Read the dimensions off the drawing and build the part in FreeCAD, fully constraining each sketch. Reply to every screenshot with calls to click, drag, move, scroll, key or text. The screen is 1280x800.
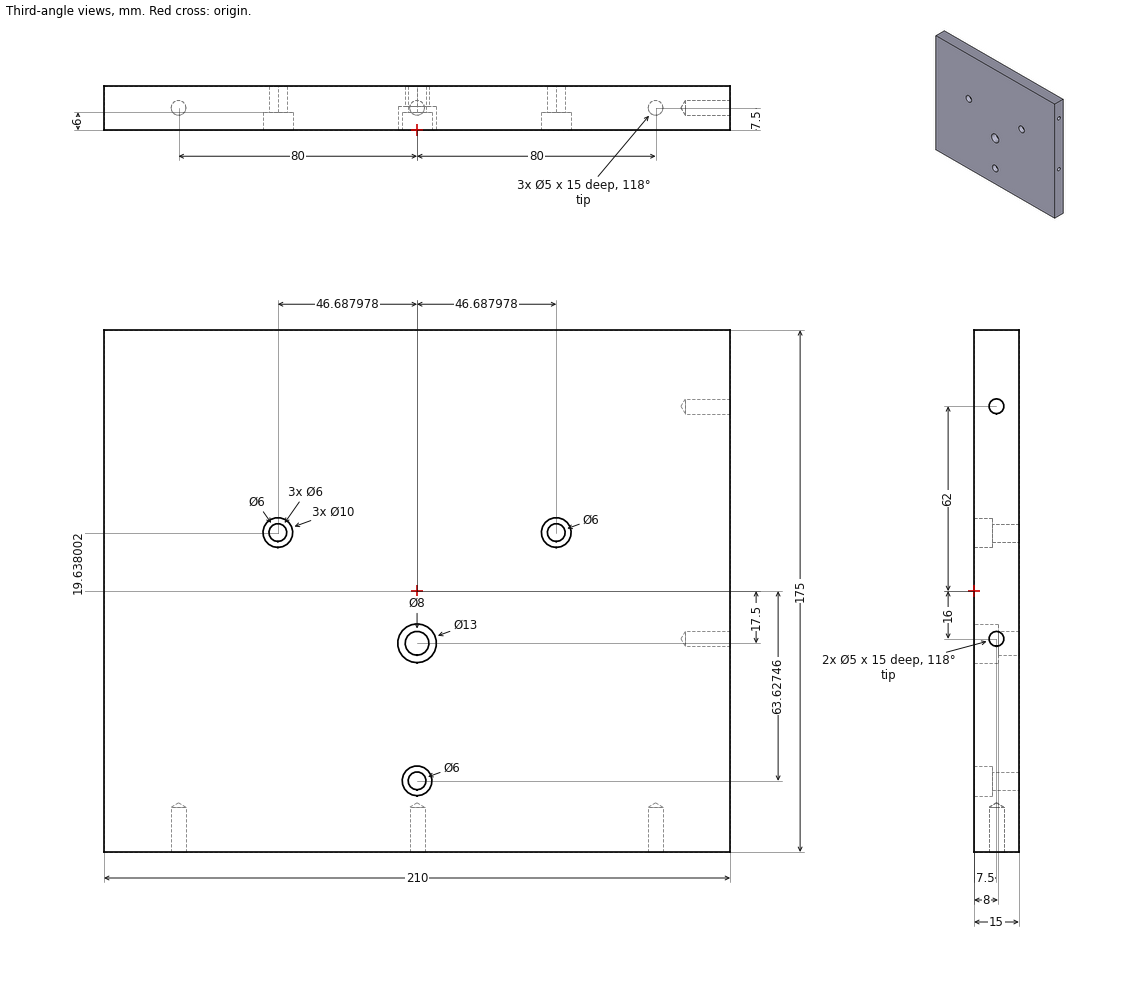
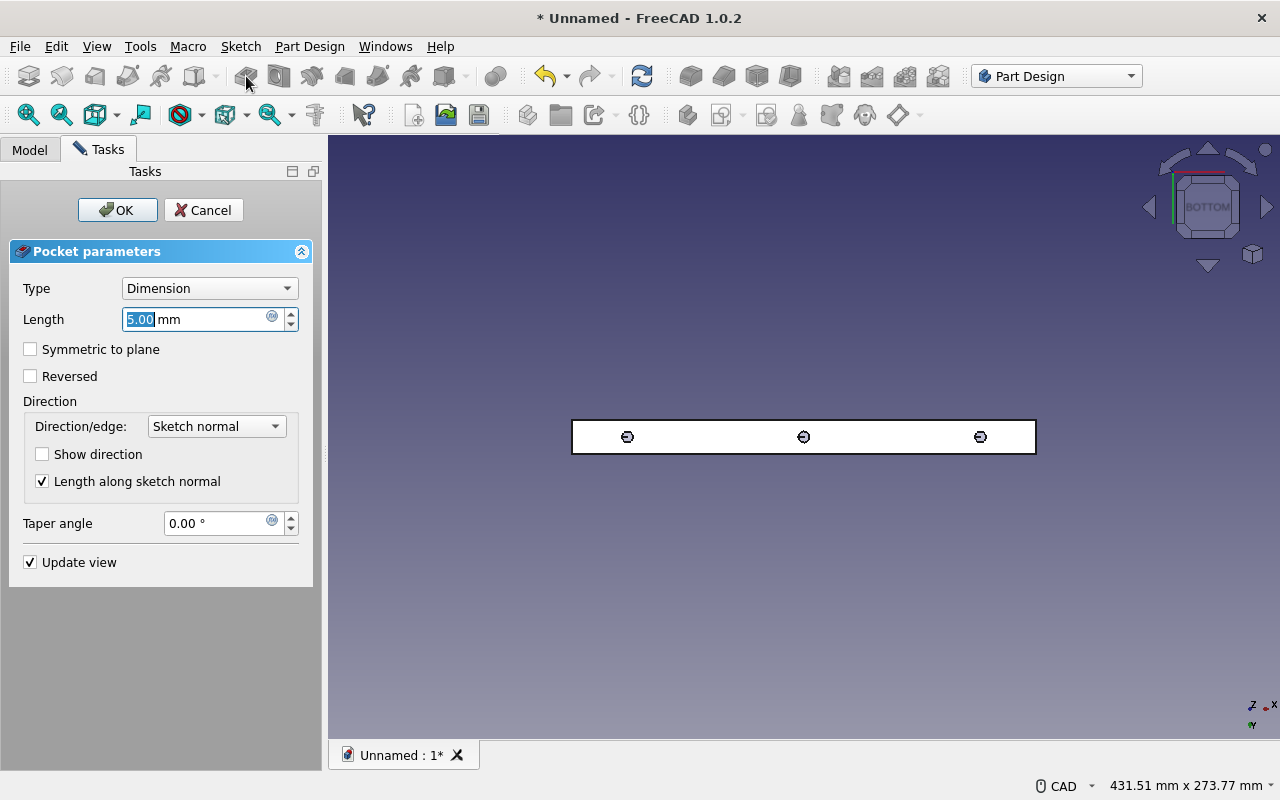
text(8)
key(Tab)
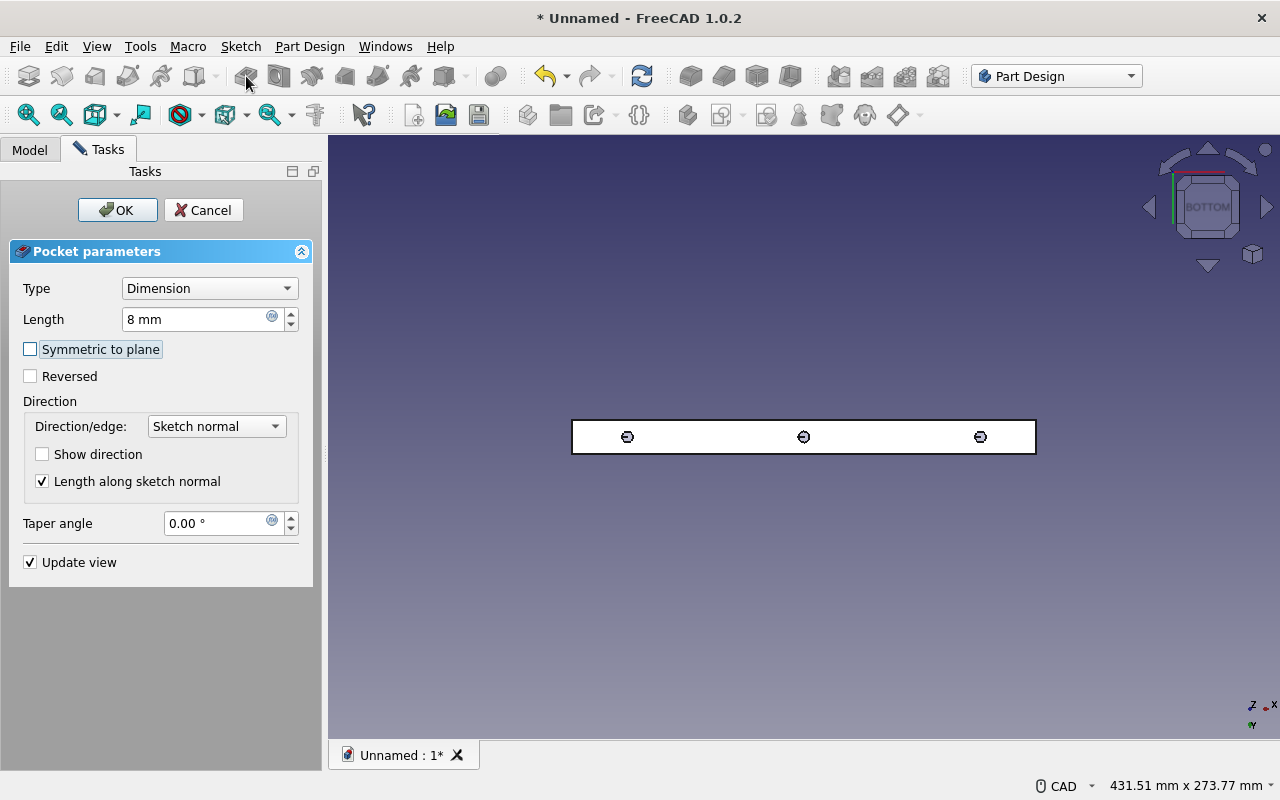
click(118, 210)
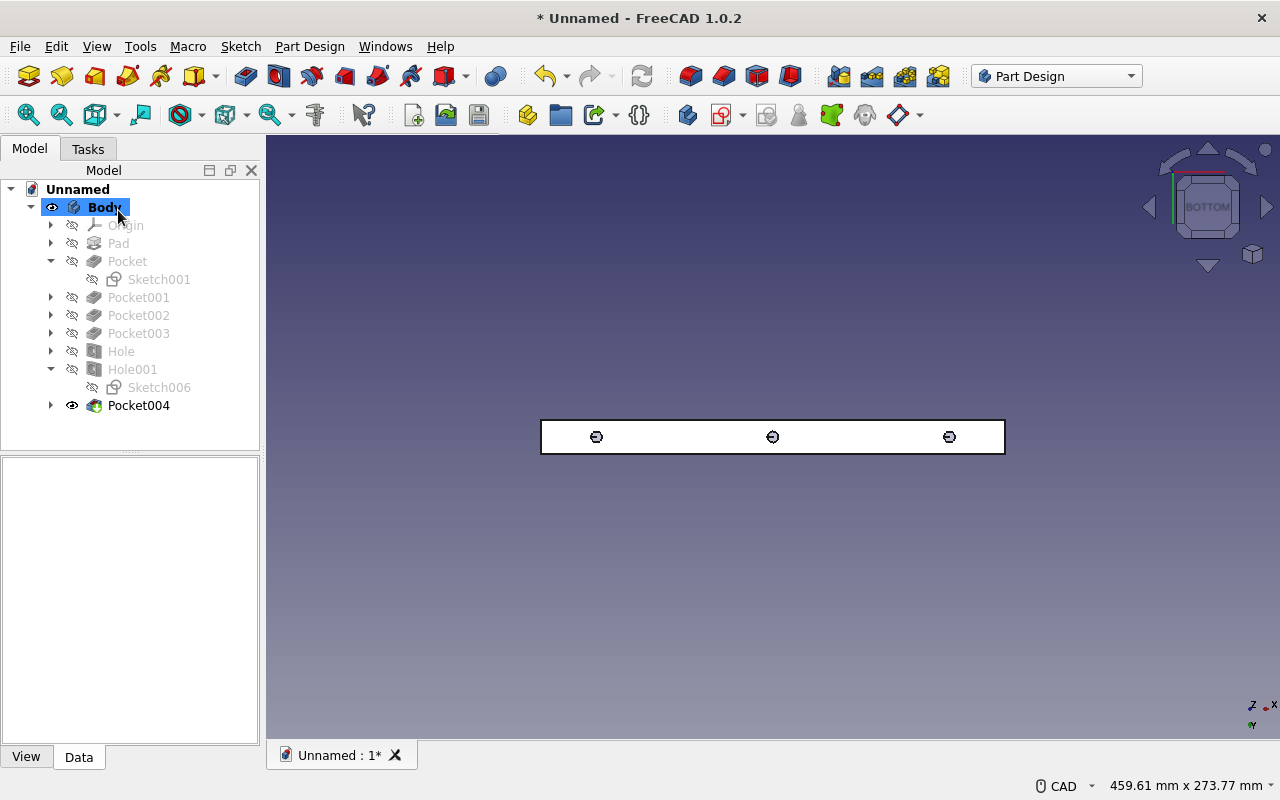
click(720, 116)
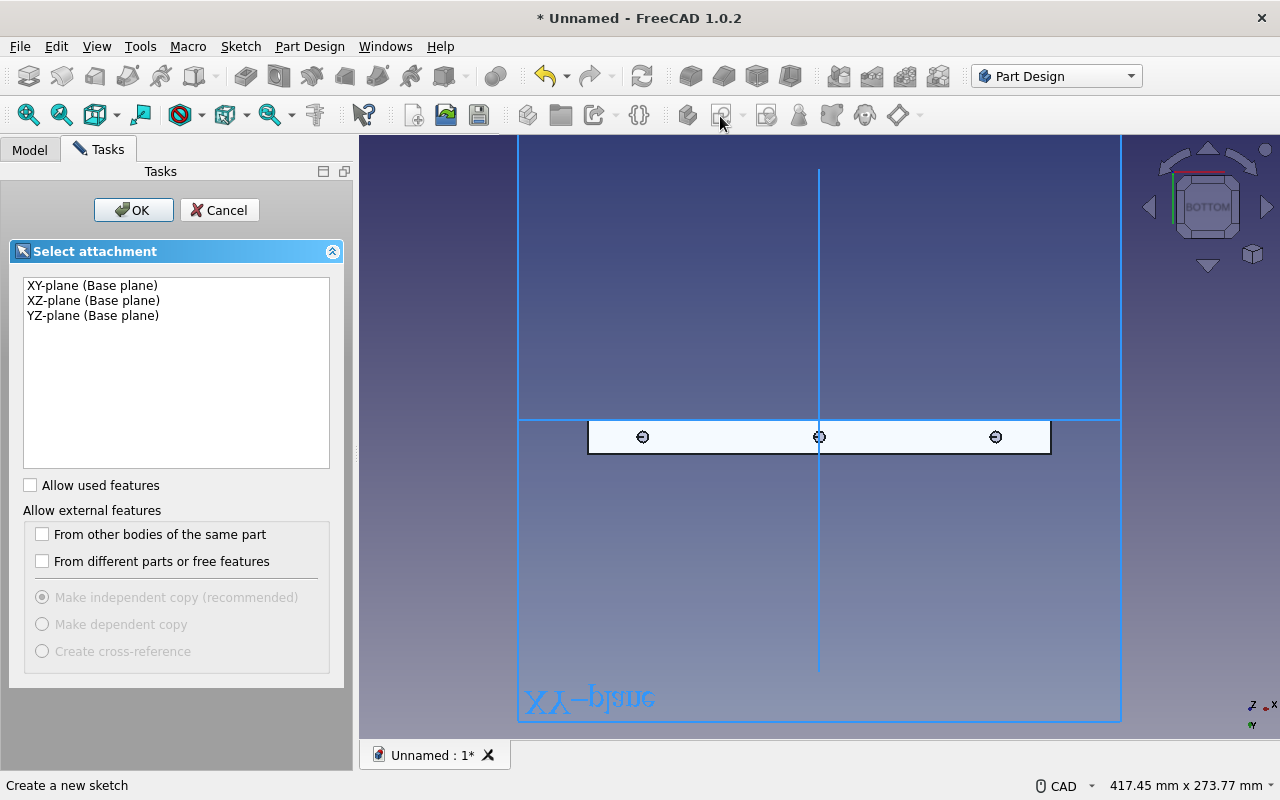
click(84, 300)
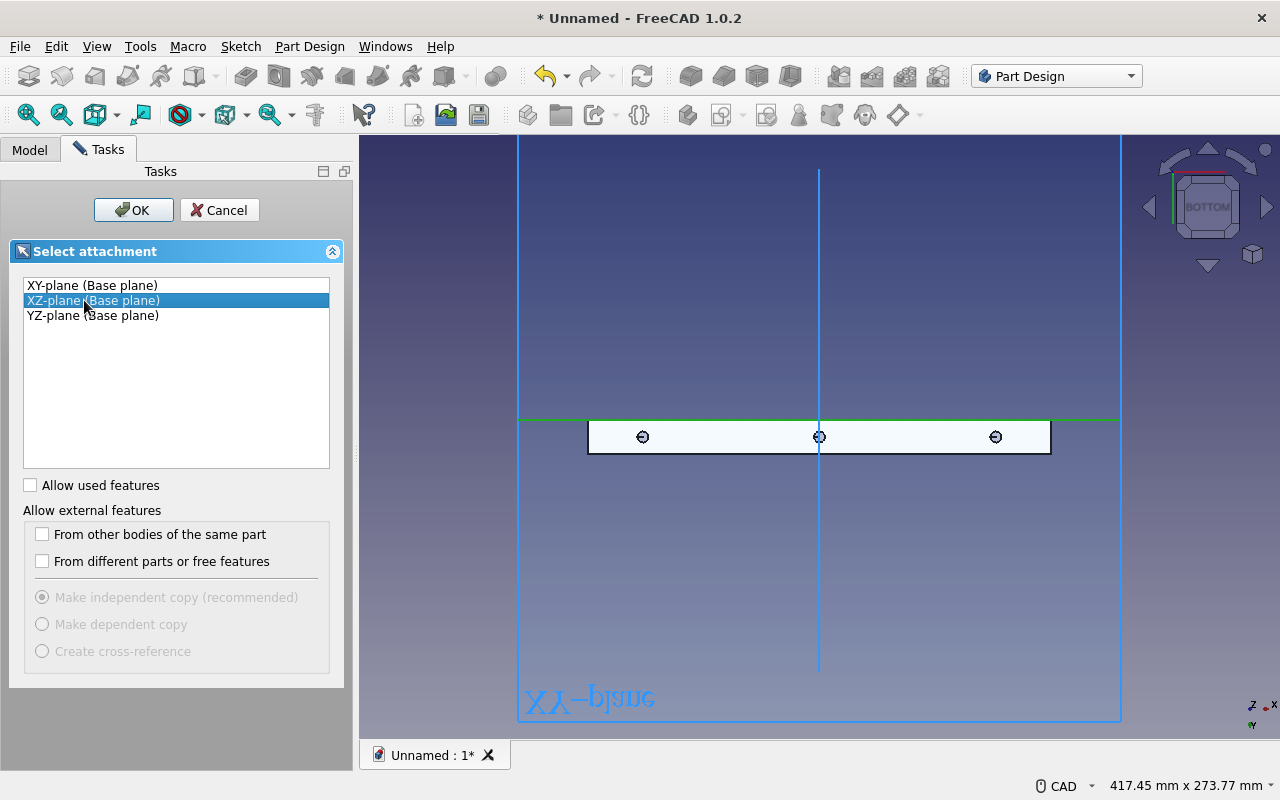
click(134, 210)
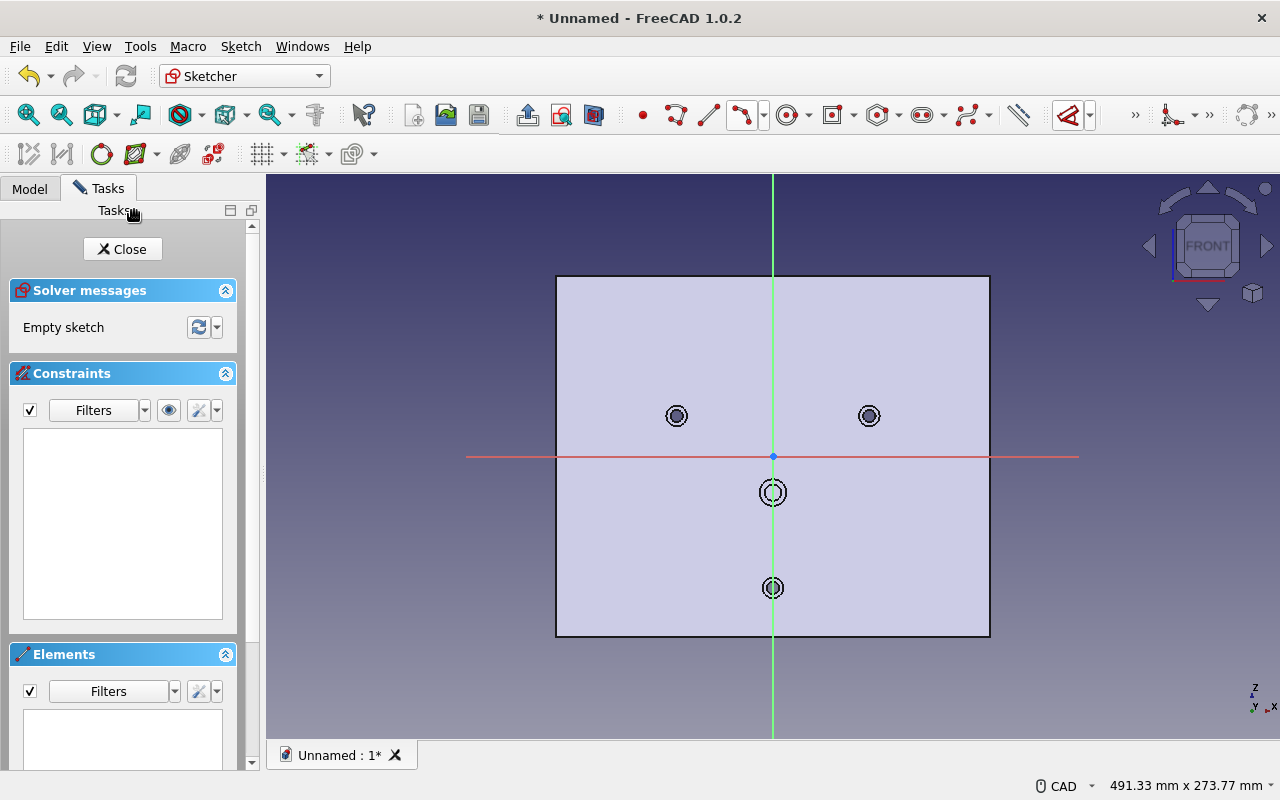
scroll(777, 495, up, 15)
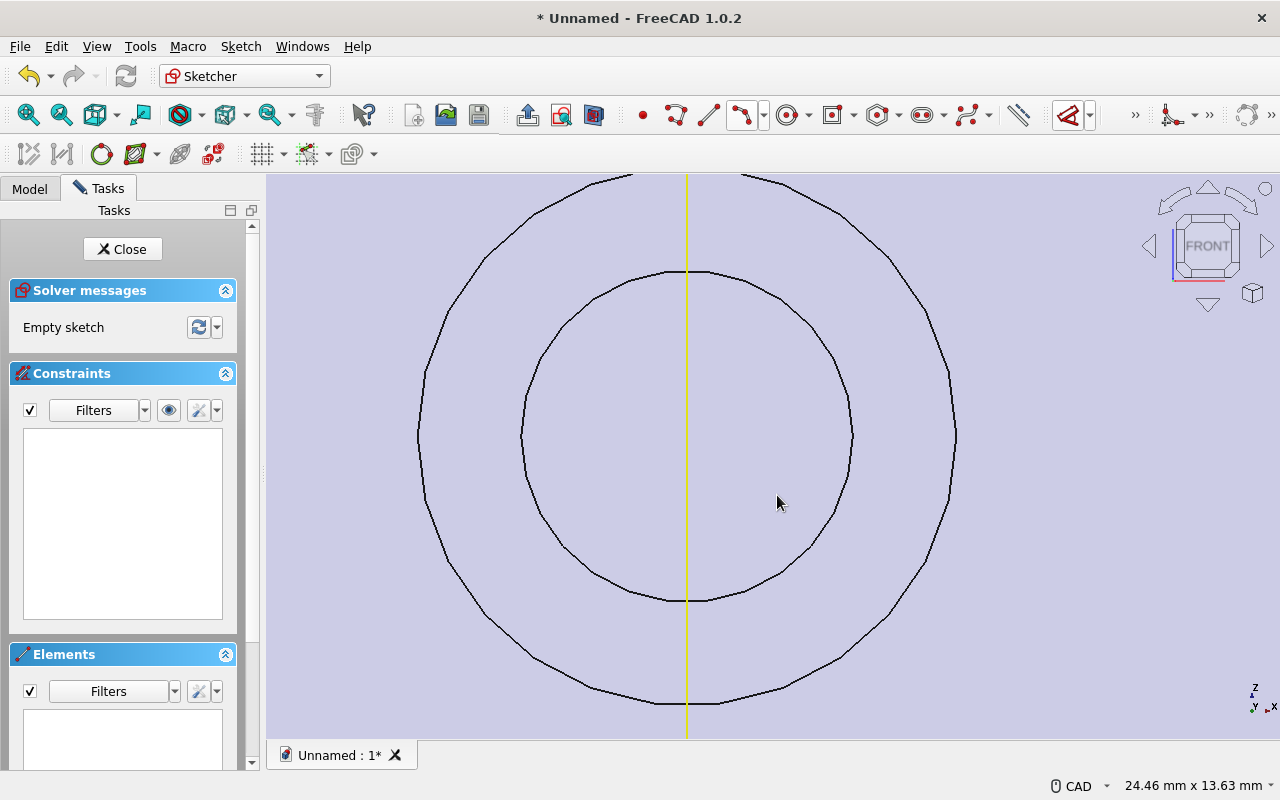
click(786, 116)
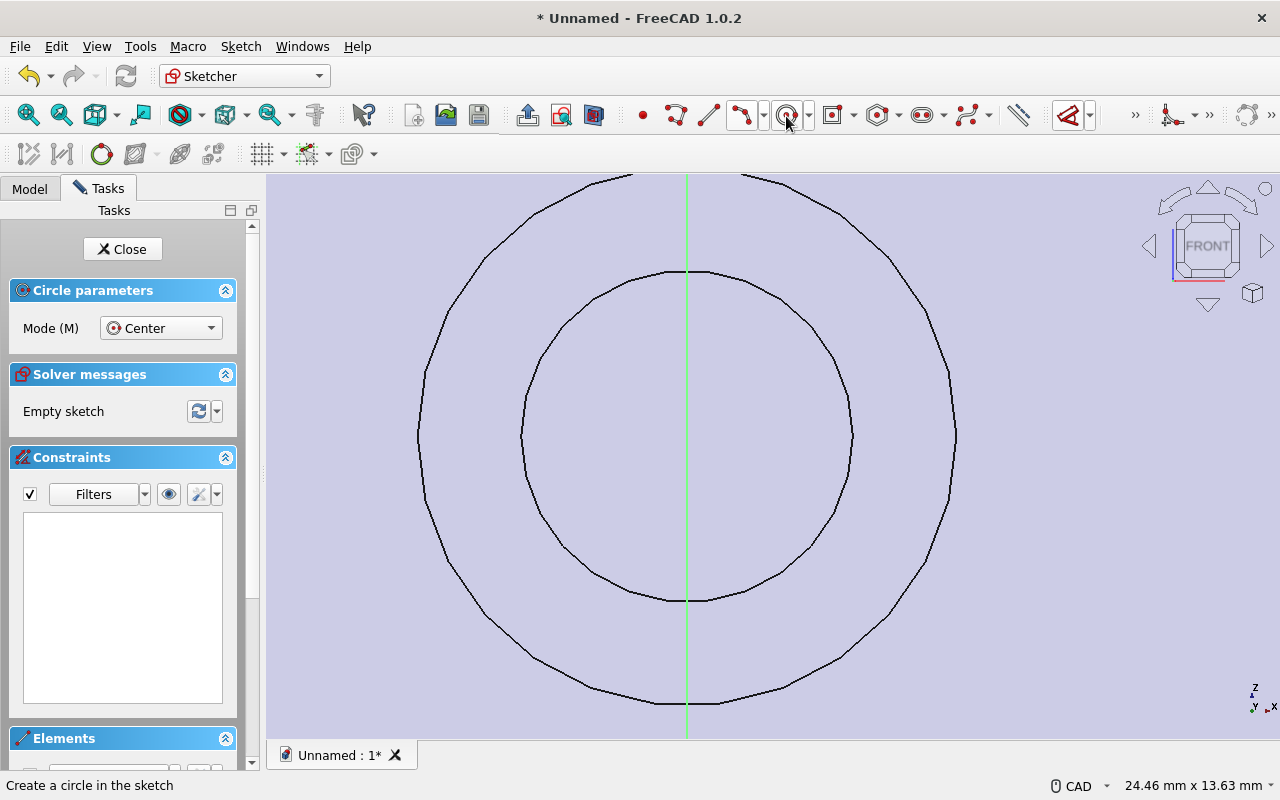
click(687, 436)
click(804, 319)
key(Escape)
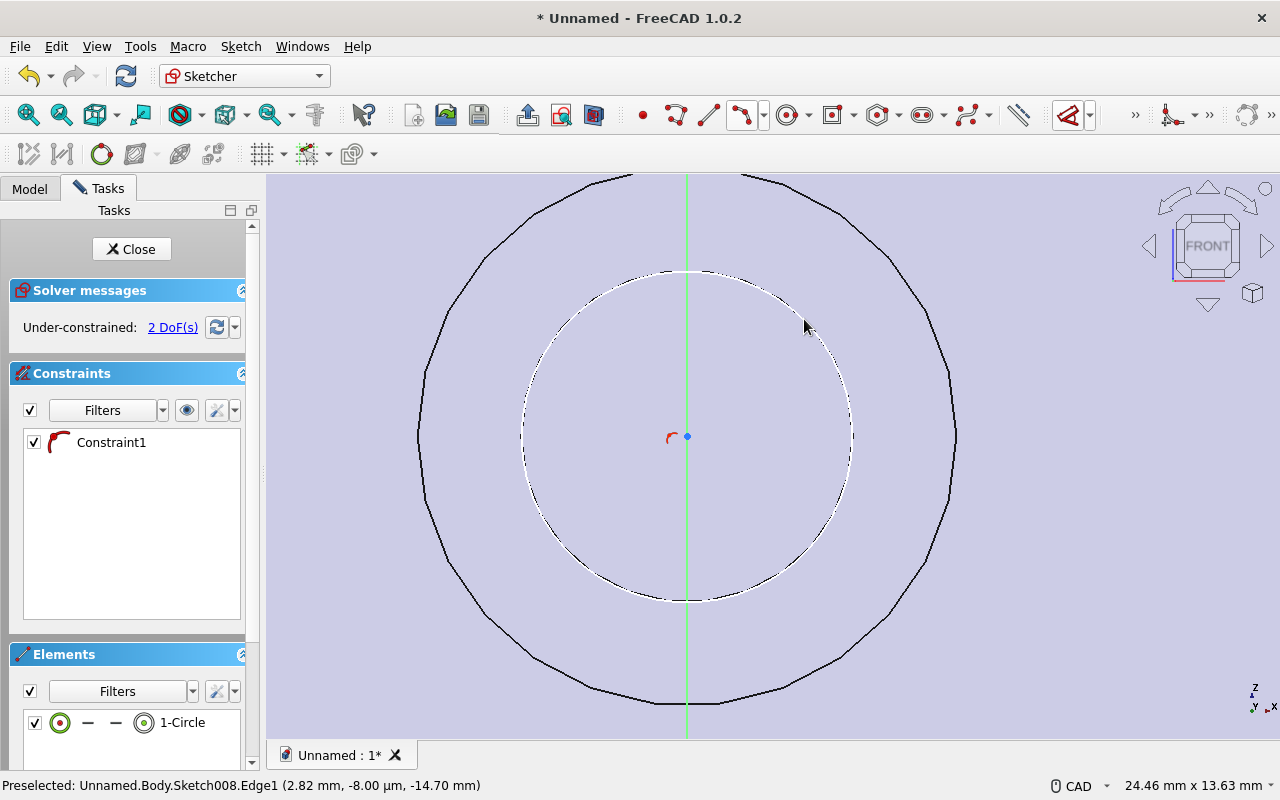
click(804, 320)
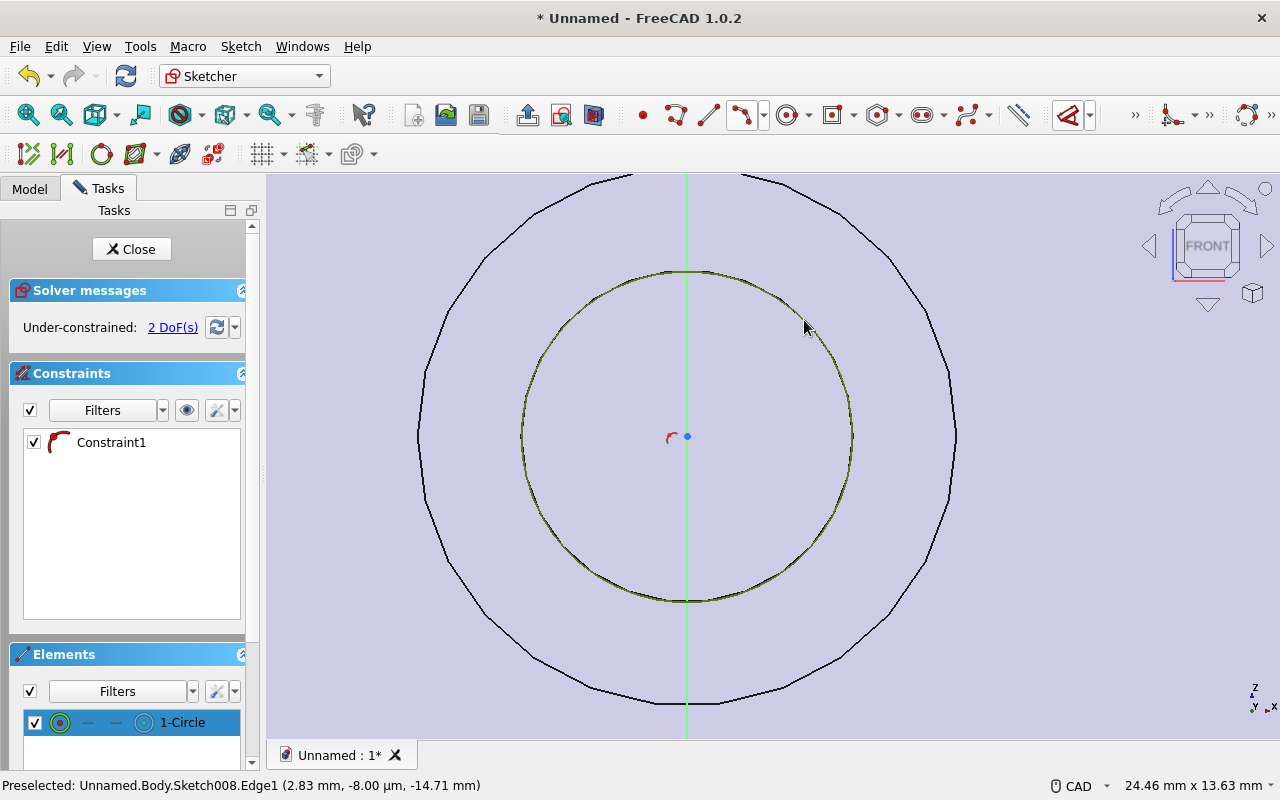
click(1090, 116)